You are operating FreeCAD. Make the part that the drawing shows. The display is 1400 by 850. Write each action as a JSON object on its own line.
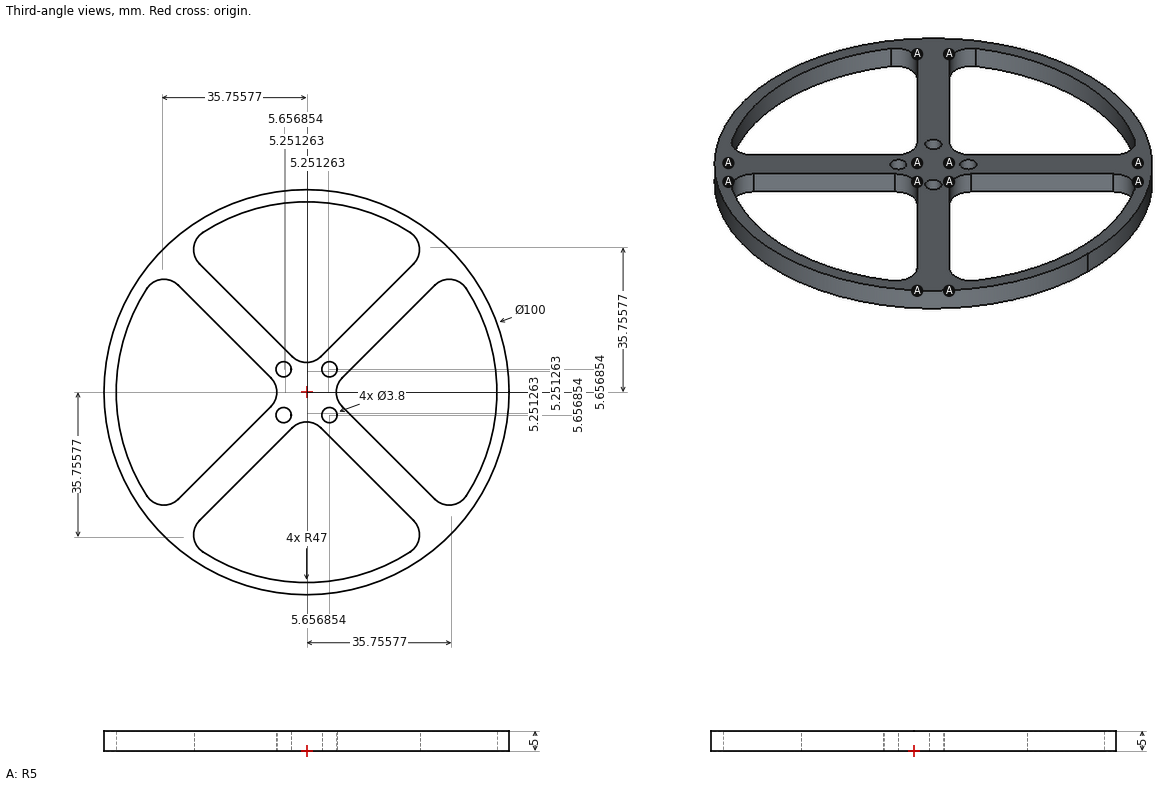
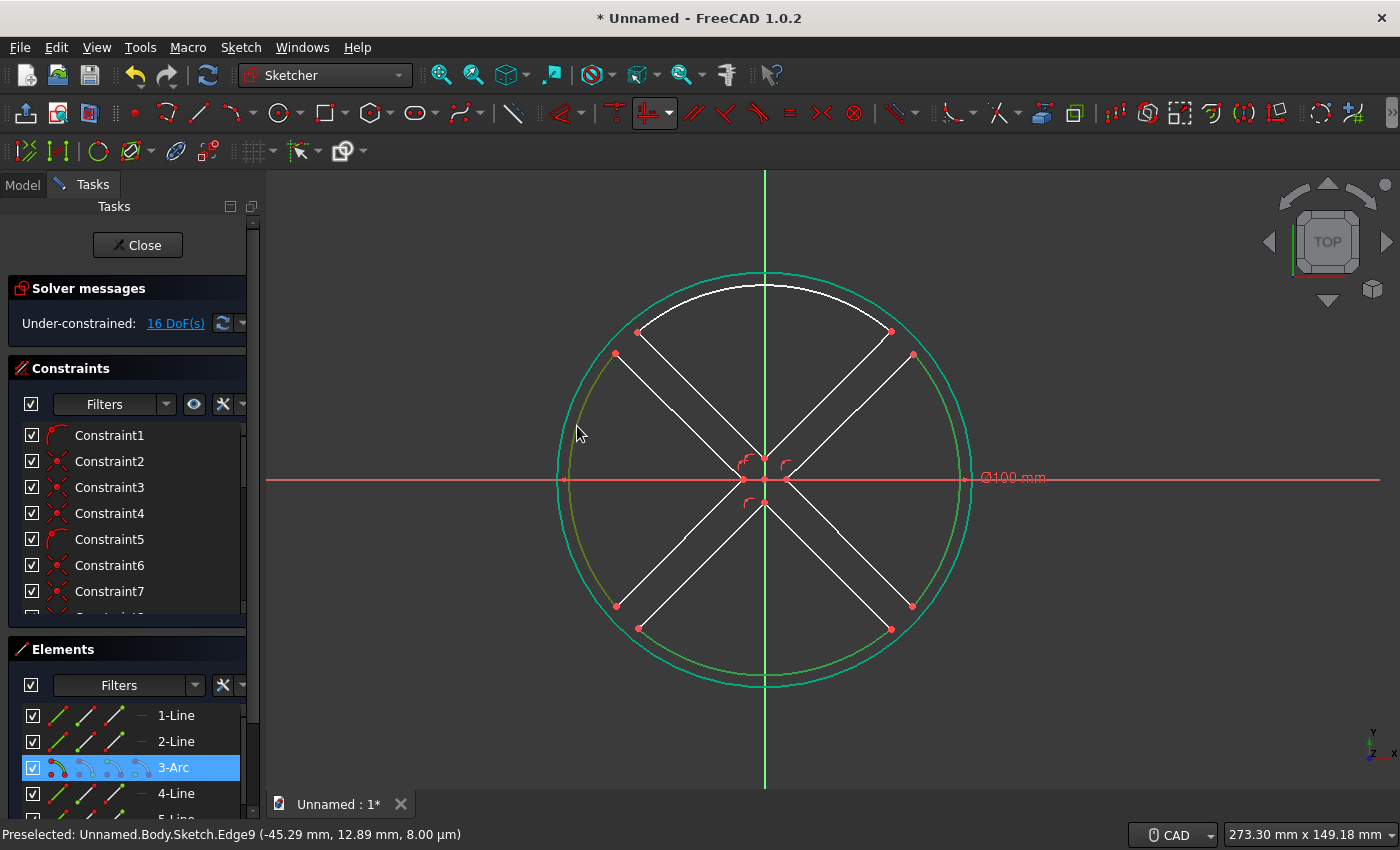
{"action": "left_click", "coordinate": [819, 293]}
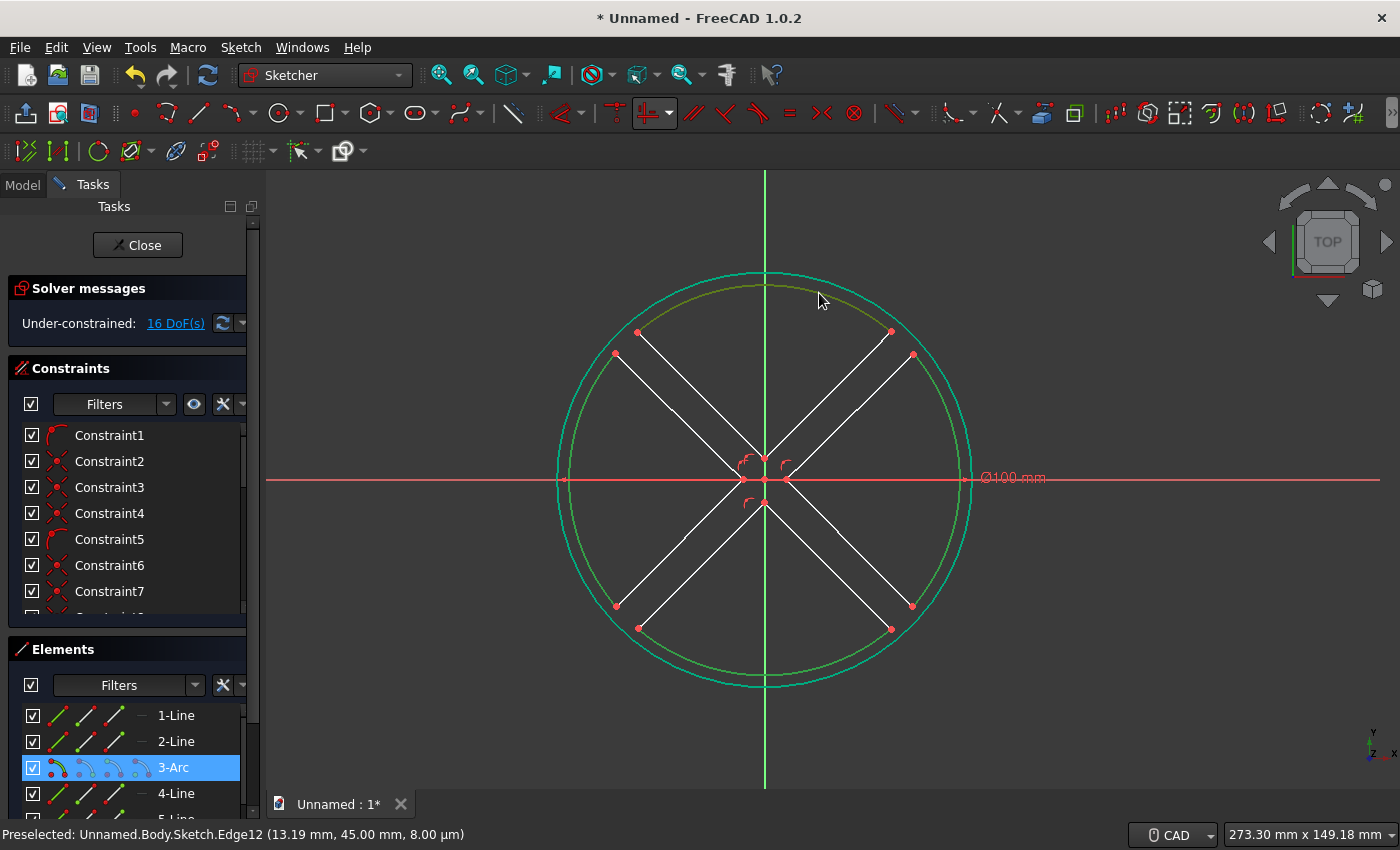
{"action": "left_click", "coordinate": [790, 114]}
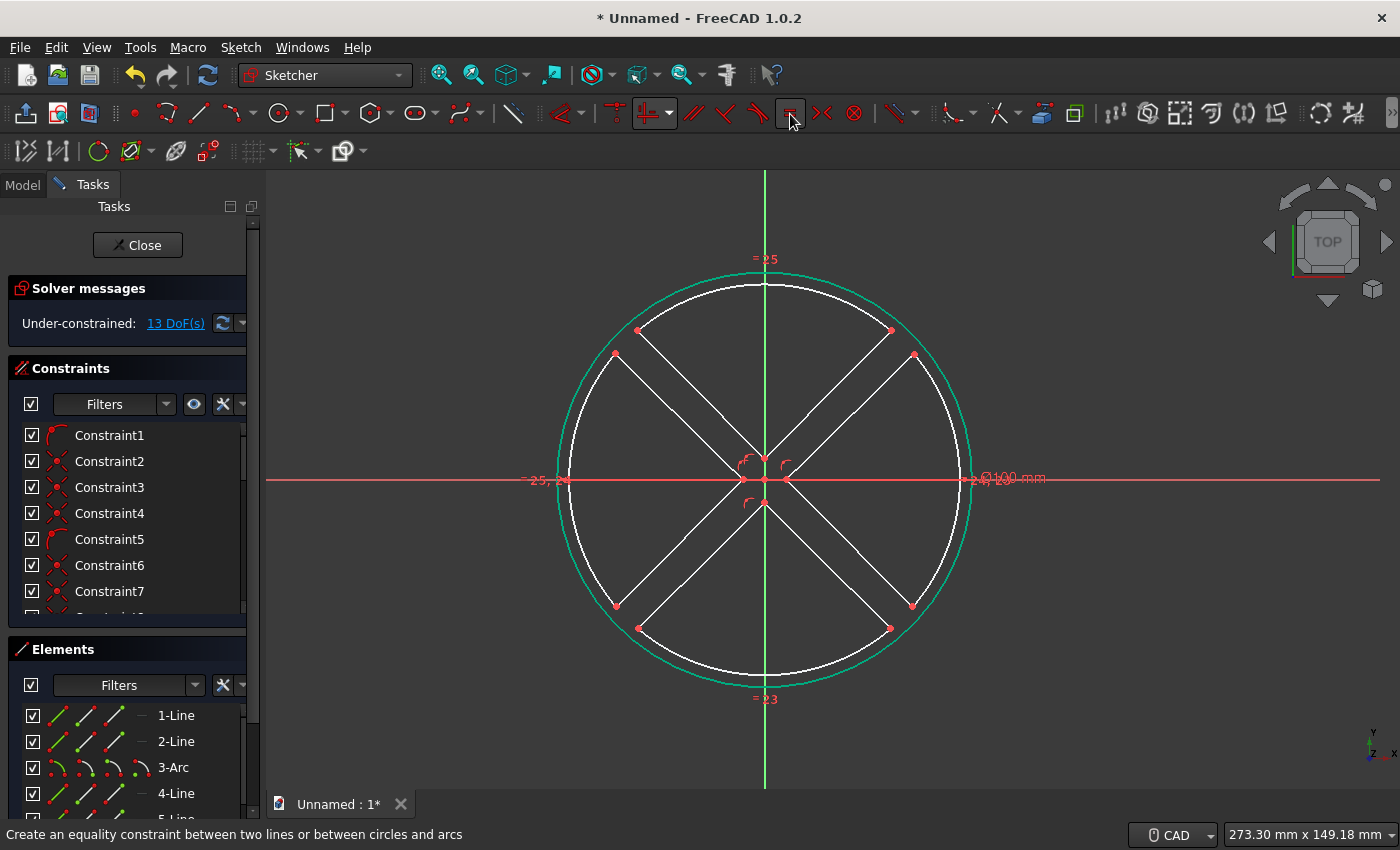
{"action": "left_click", "coordinate": [710, 668]}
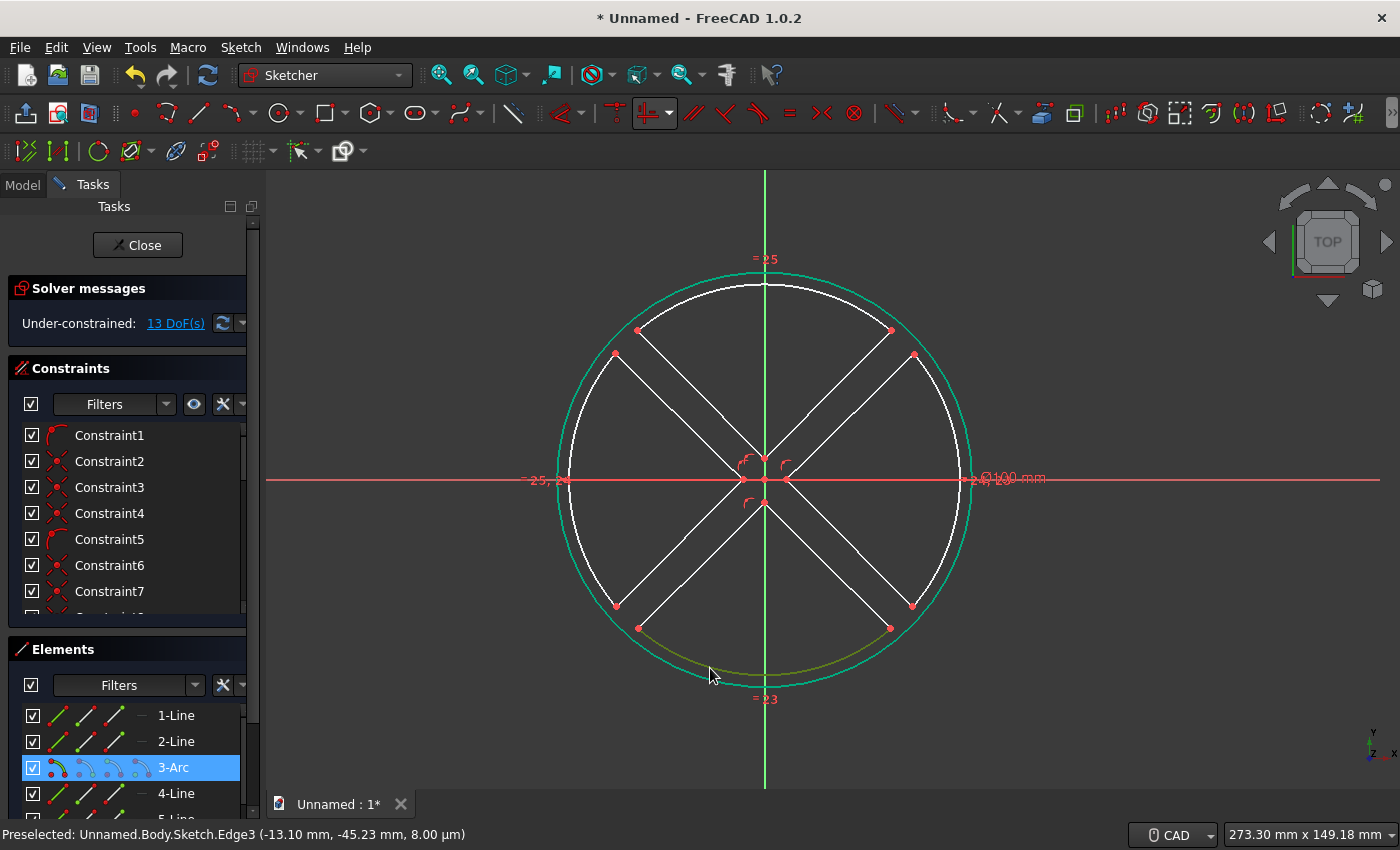
{"action": "left_click", "coordinate": [584, 114]}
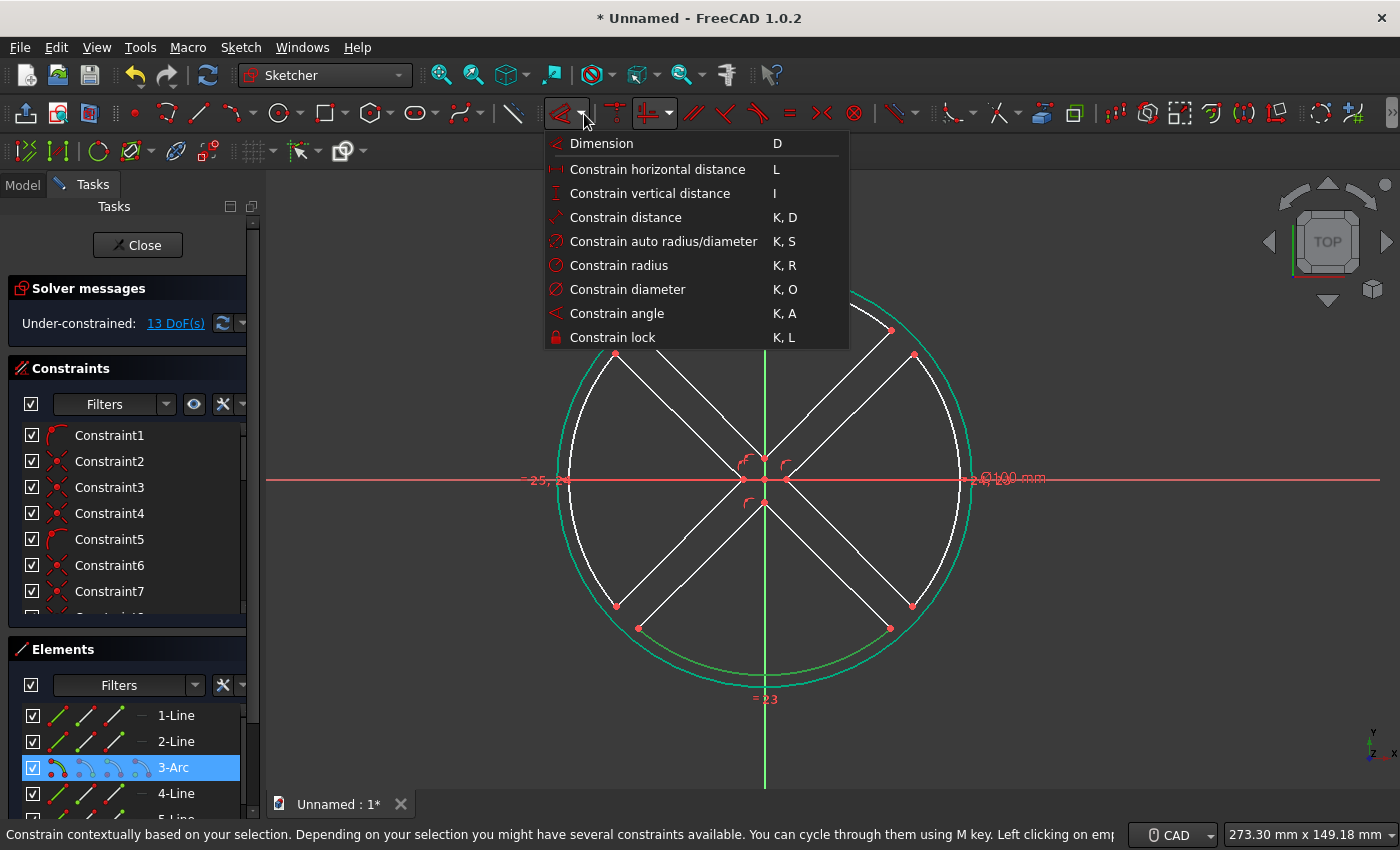
{"action": "left_click", "coordinate": [697, 265]}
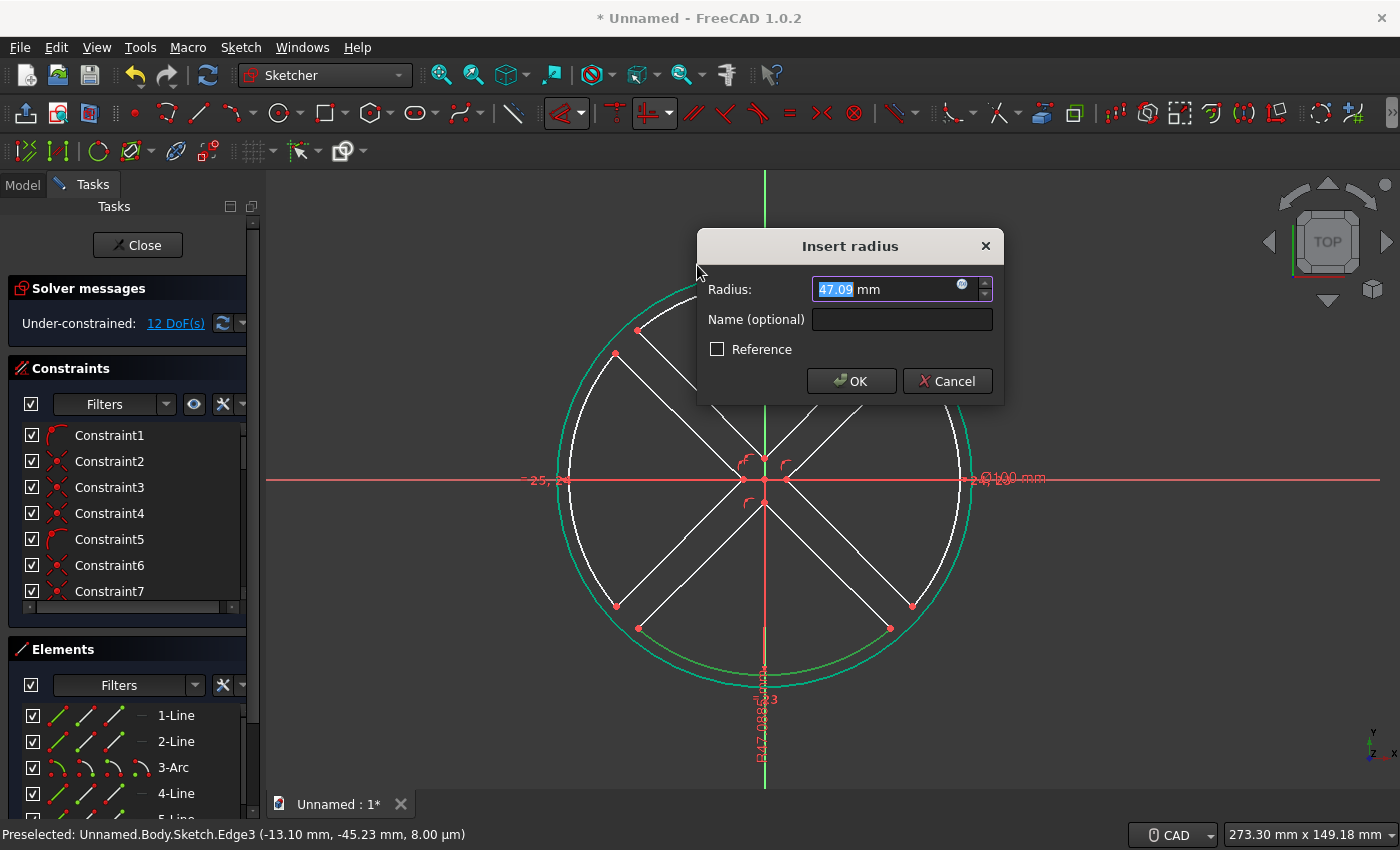
{"action": "type", "text": "47"}
{"action": "key", "text": "Return"}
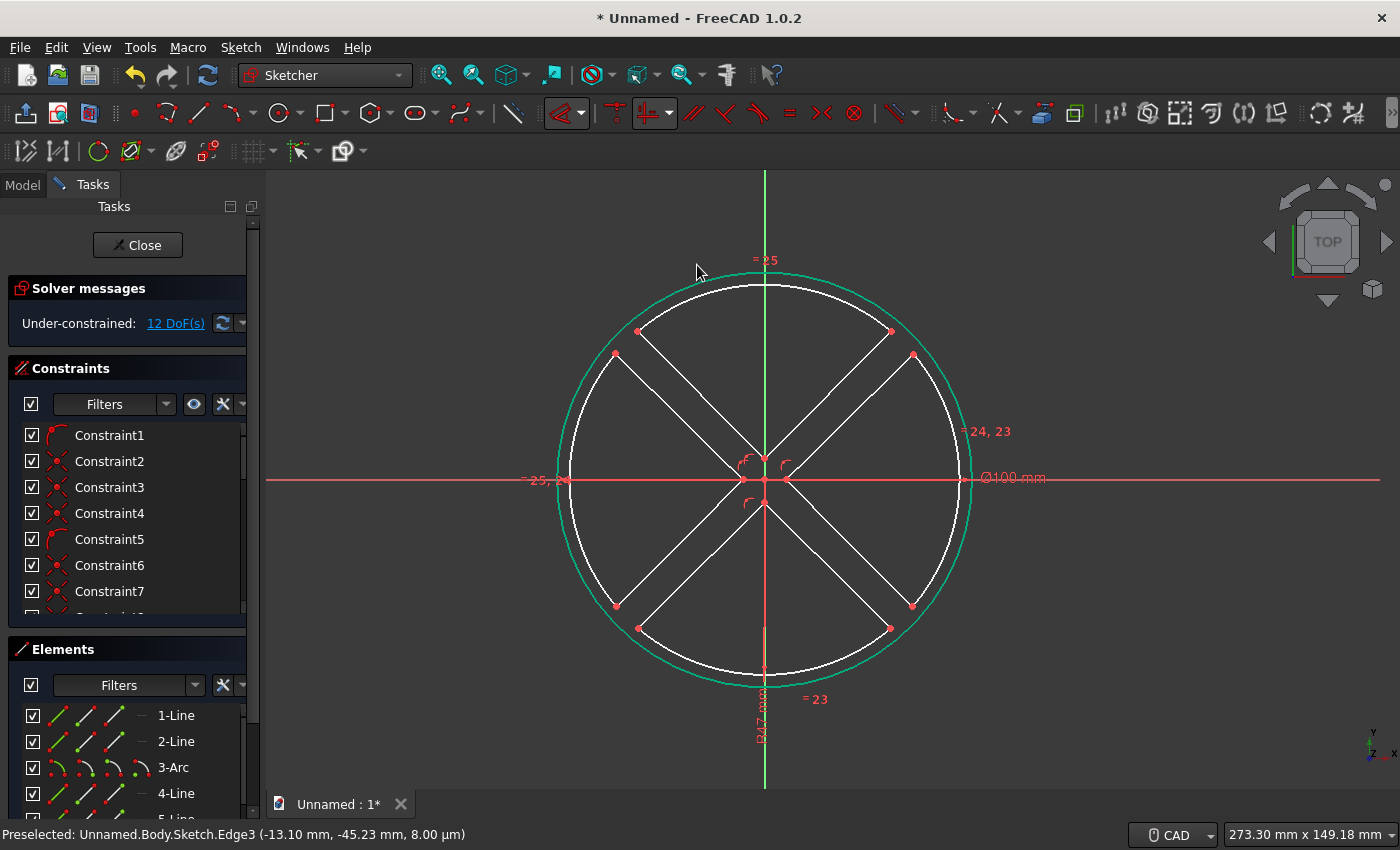
{"action": "left_click", "coordinate": [638, 628]}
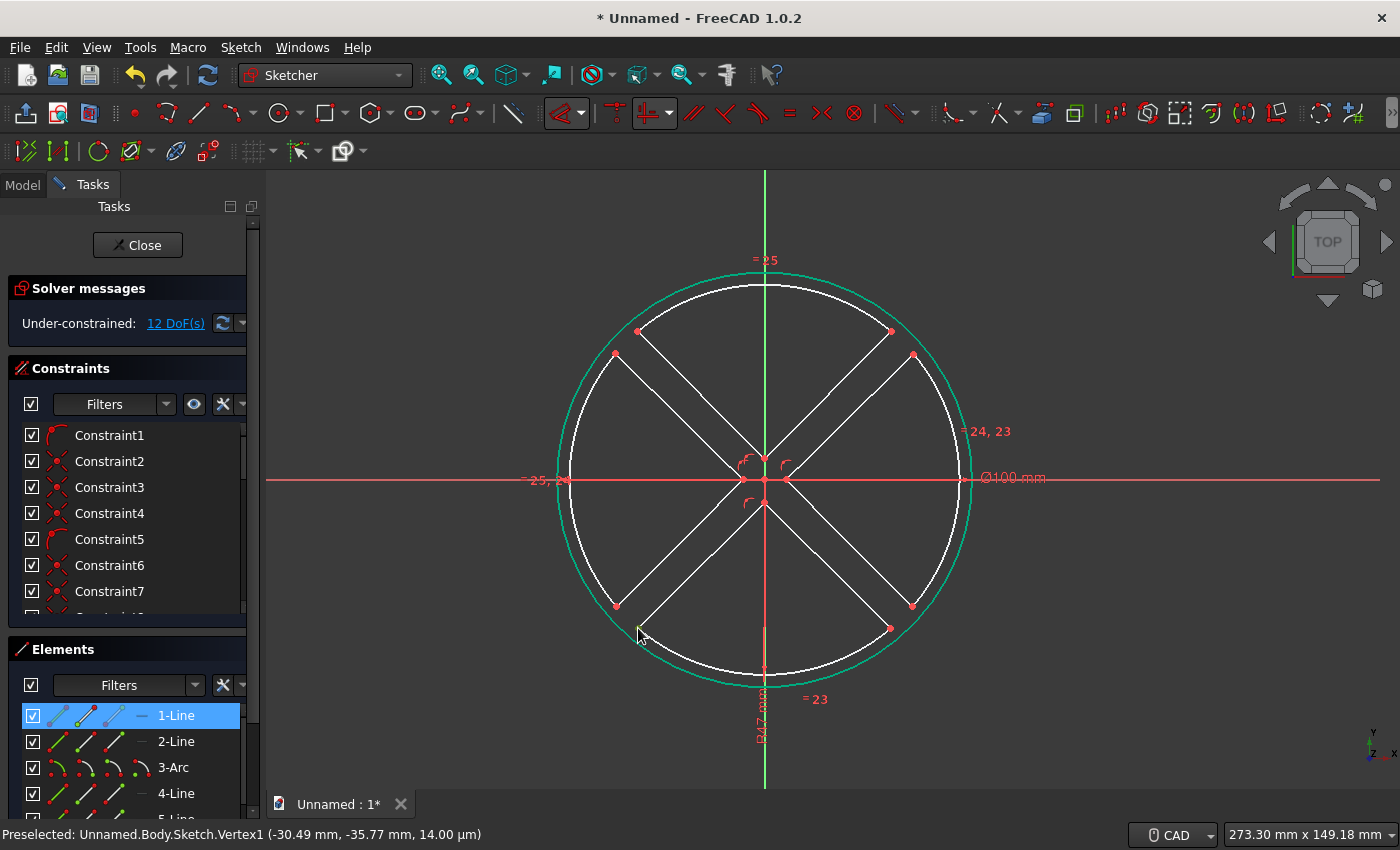
{"action": "left_click", "coordinate": [584, 114]}